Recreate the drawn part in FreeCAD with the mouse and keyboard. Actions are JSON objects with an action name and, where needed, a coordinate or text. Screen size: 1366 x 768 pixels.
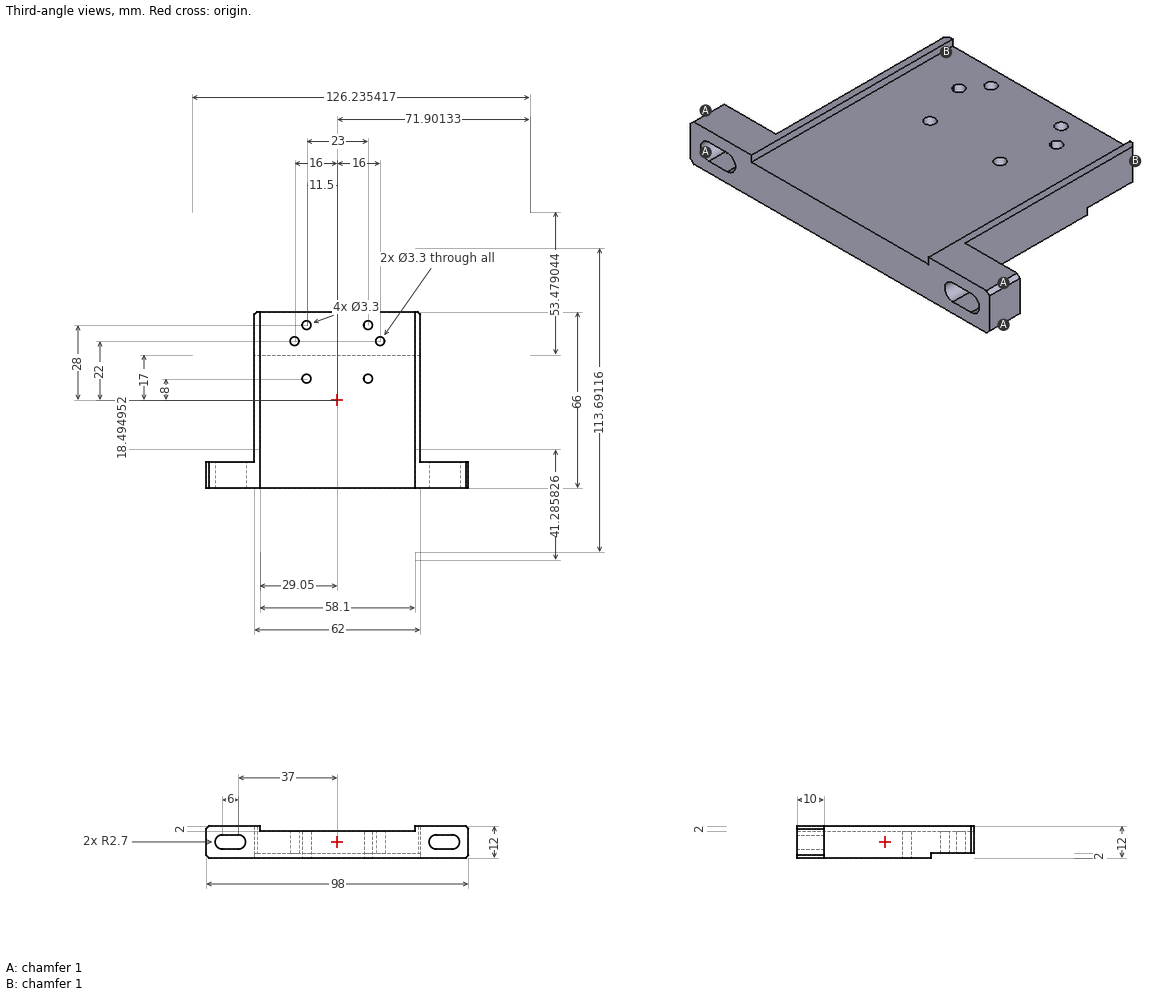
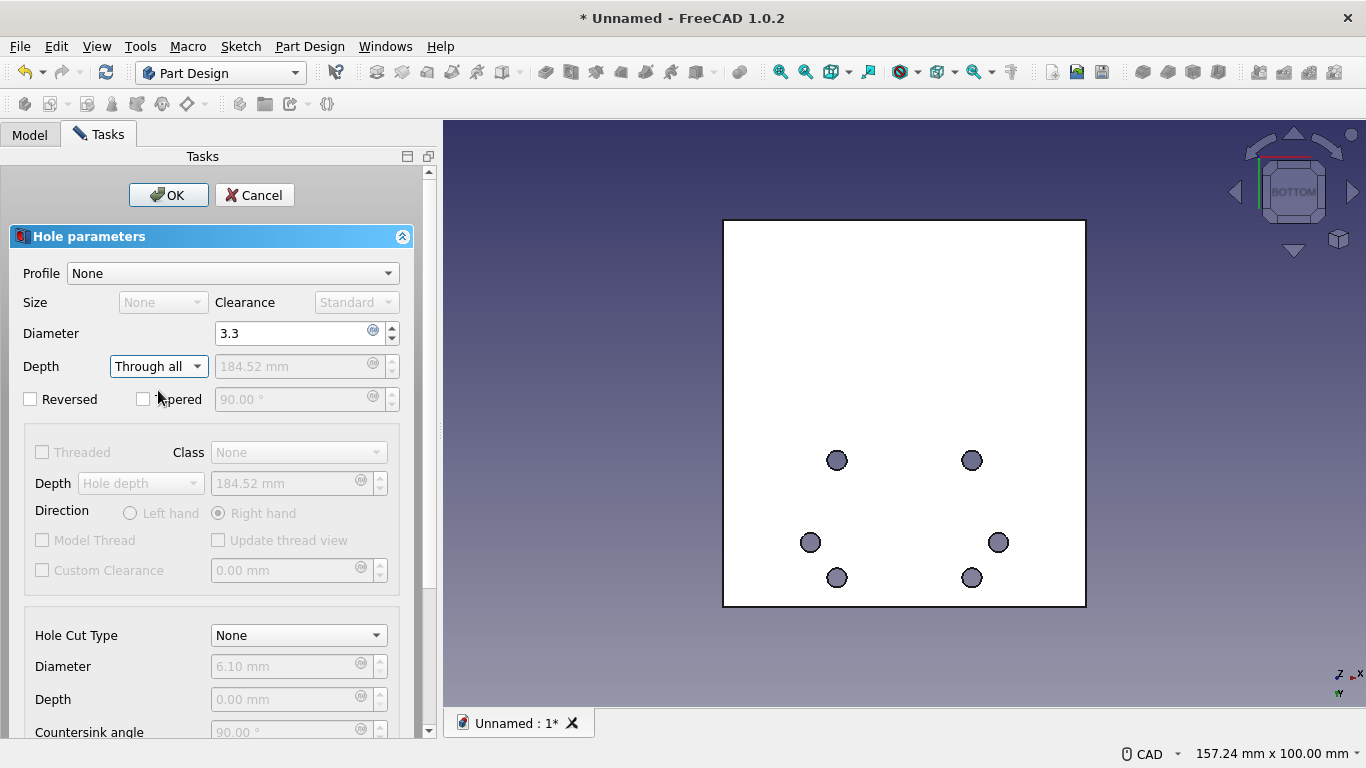
{"action": "left_click", "coordinate": [169, 195]}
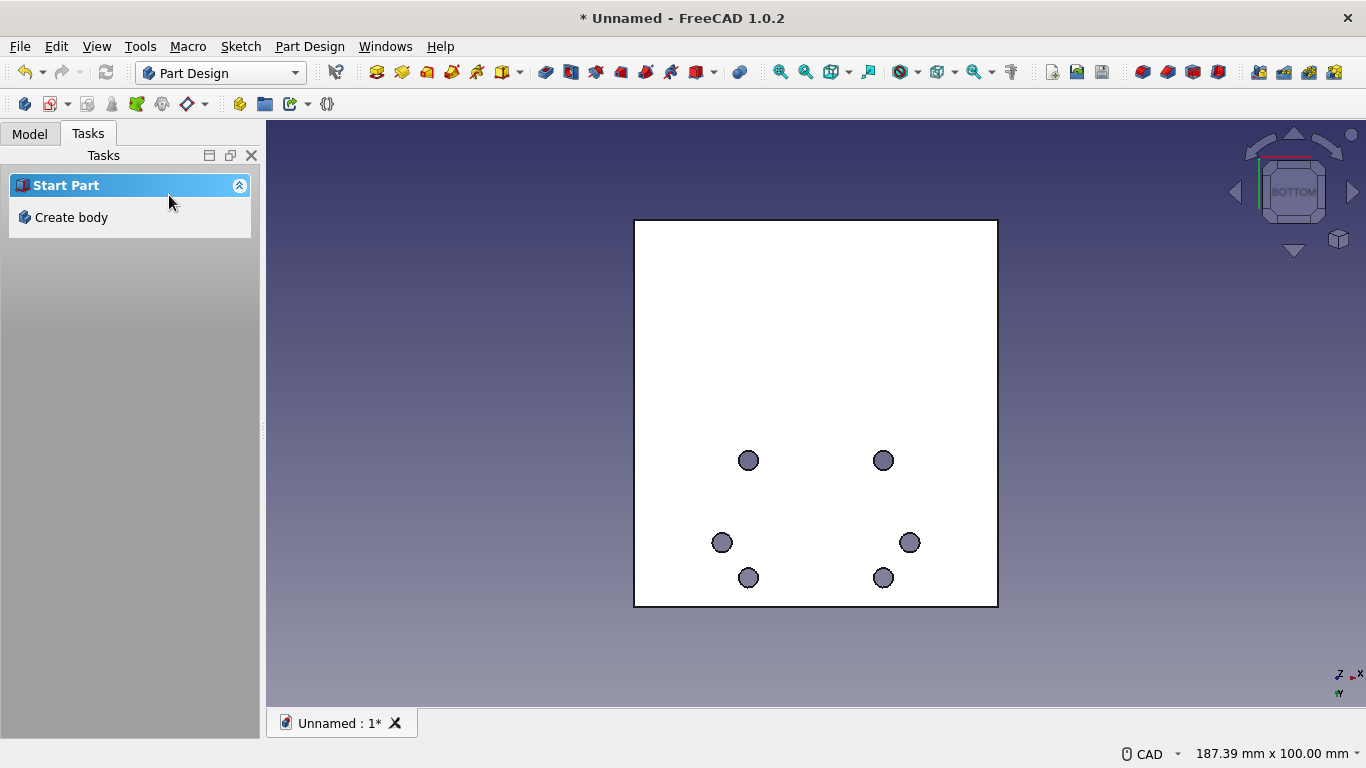
{"action": "key", "text": "0"}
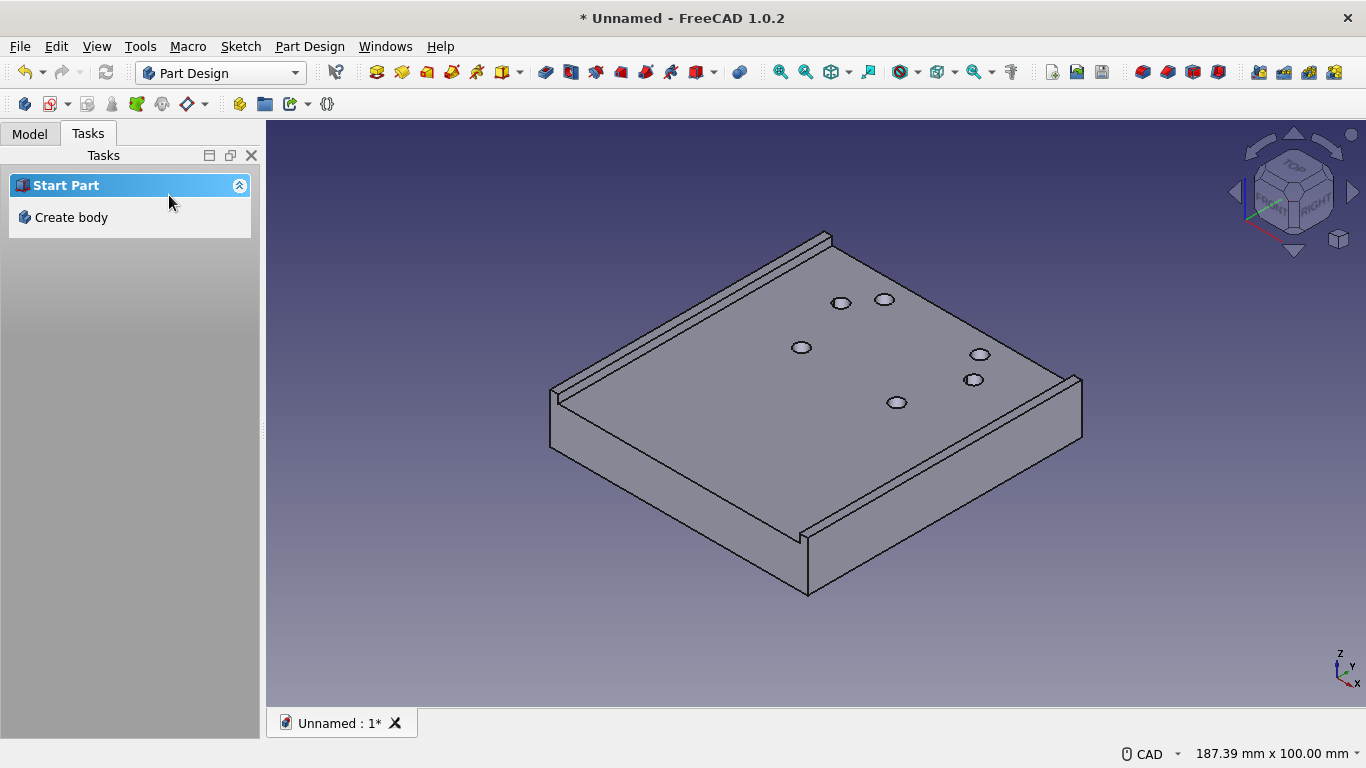
{"action": "left_click", "coordinate": [789, 563]}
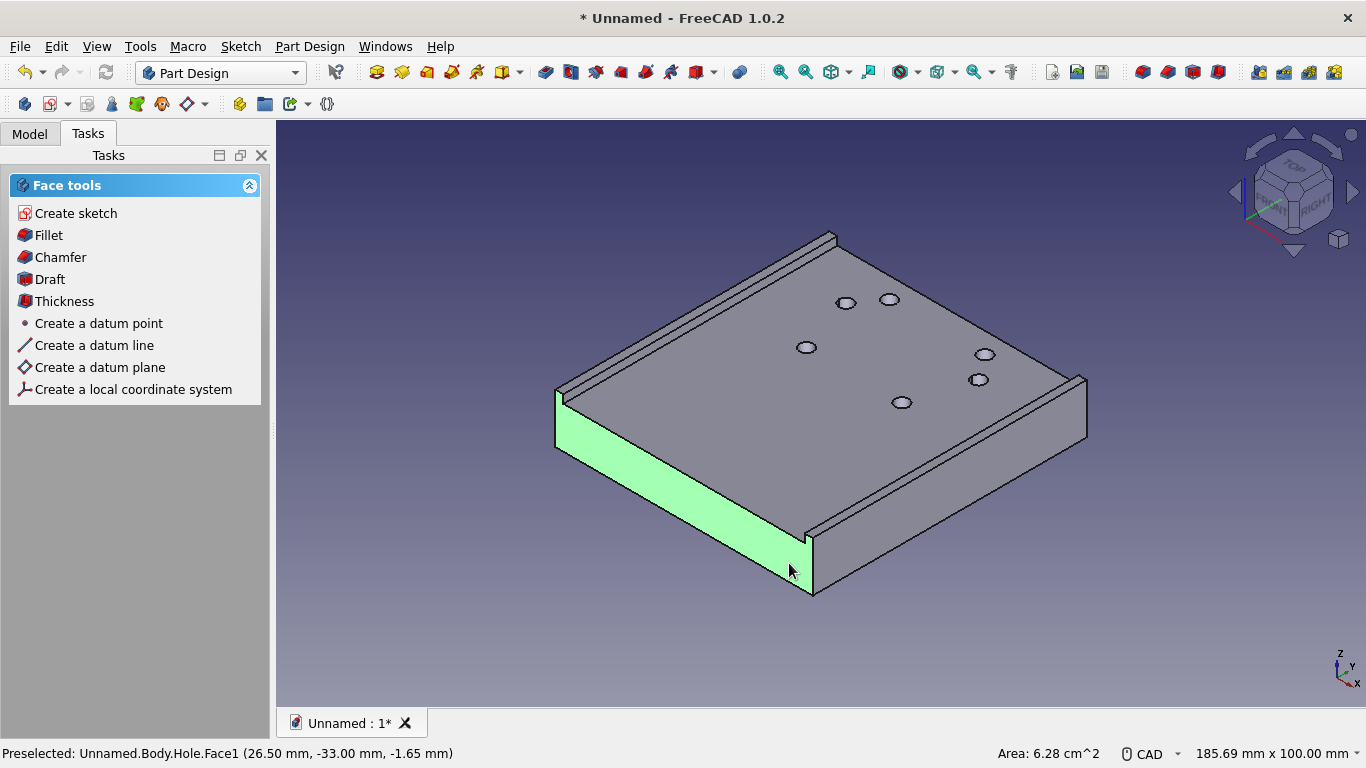
{"action": "left_click", "coordinate": [50, 104]}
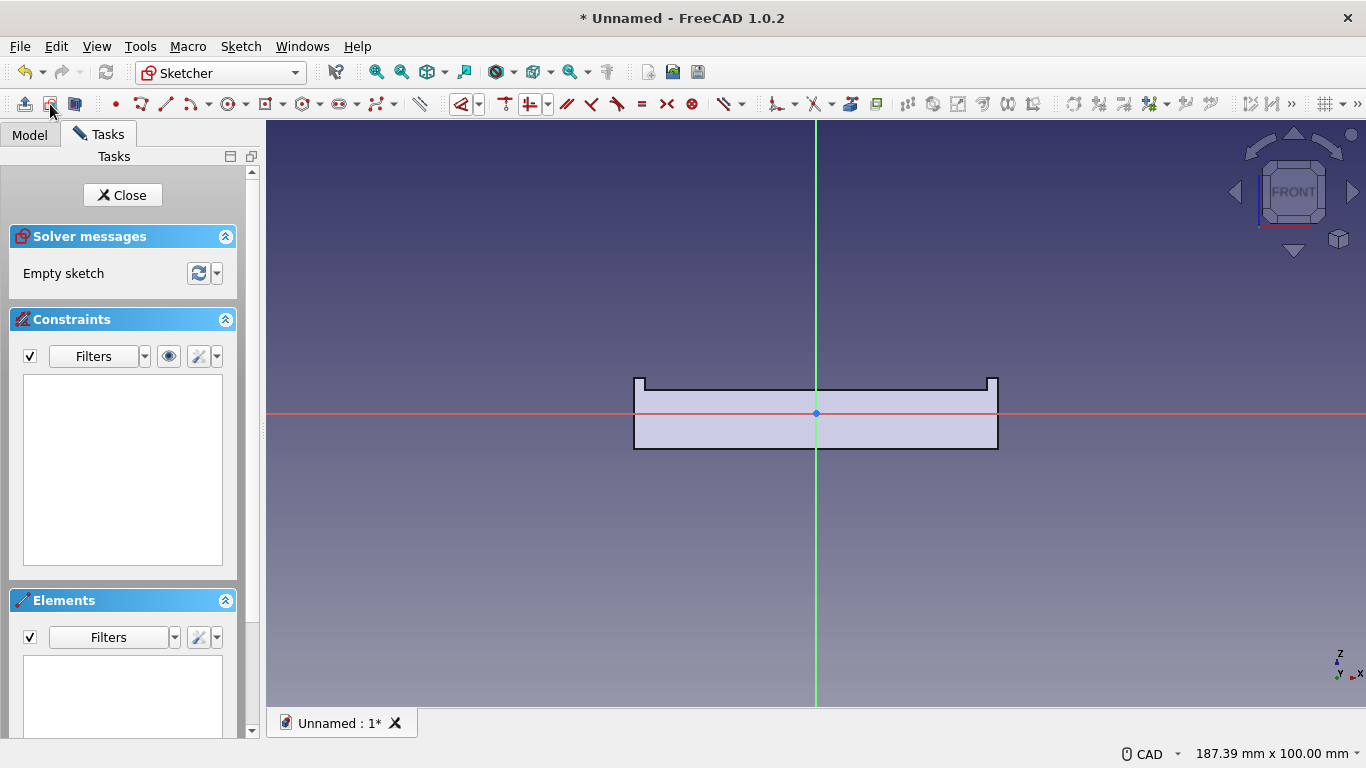
{"action": "left_click", "coordinate": [264, 104]}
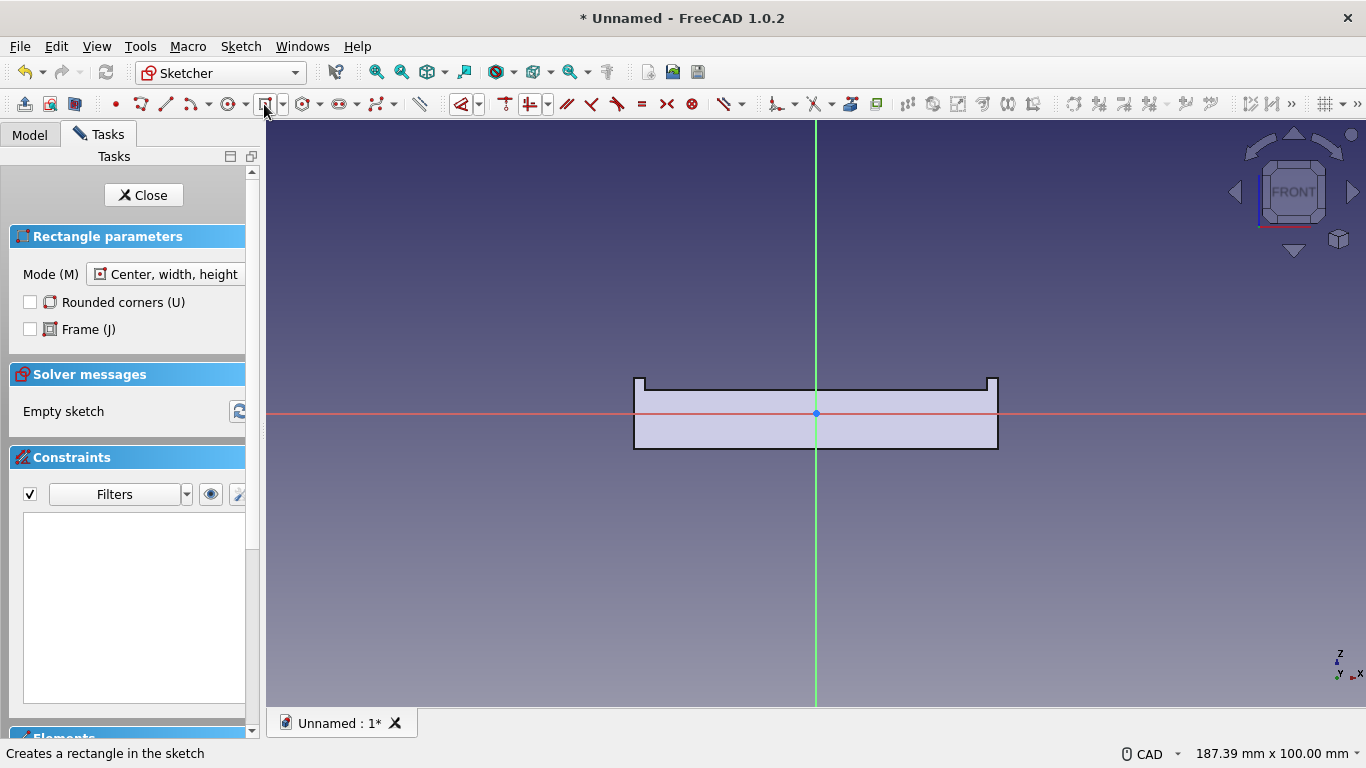
{"action": "left_click", "coordinate": [816, 413]}
{"action": "mouse_move", "coordinate": [1104, 378]}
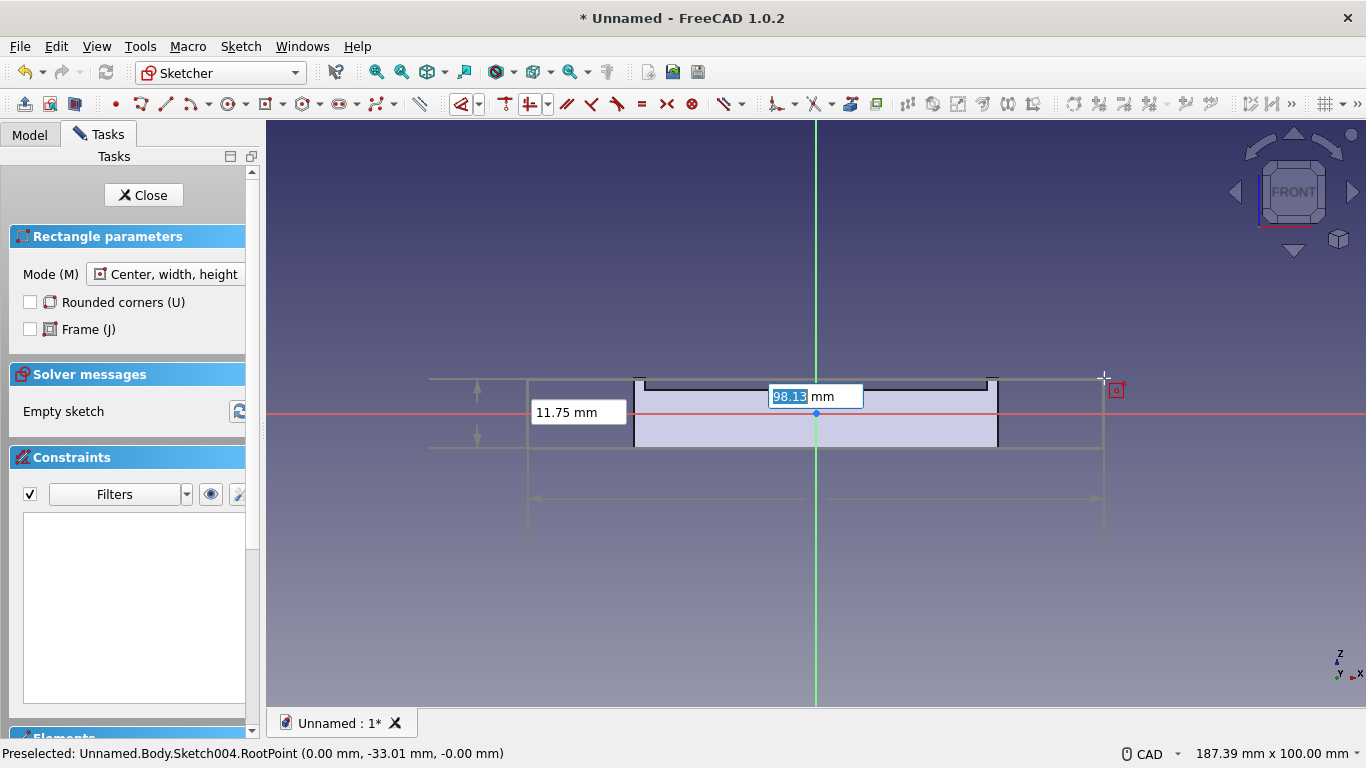
{"action": "type", "text": "98"}
{"action": "key", "text": "Tab"}
{"action": "type", "text": "12"}
{"action": "key", "text": "Return"}
{"action": "key", "text": "Escape"}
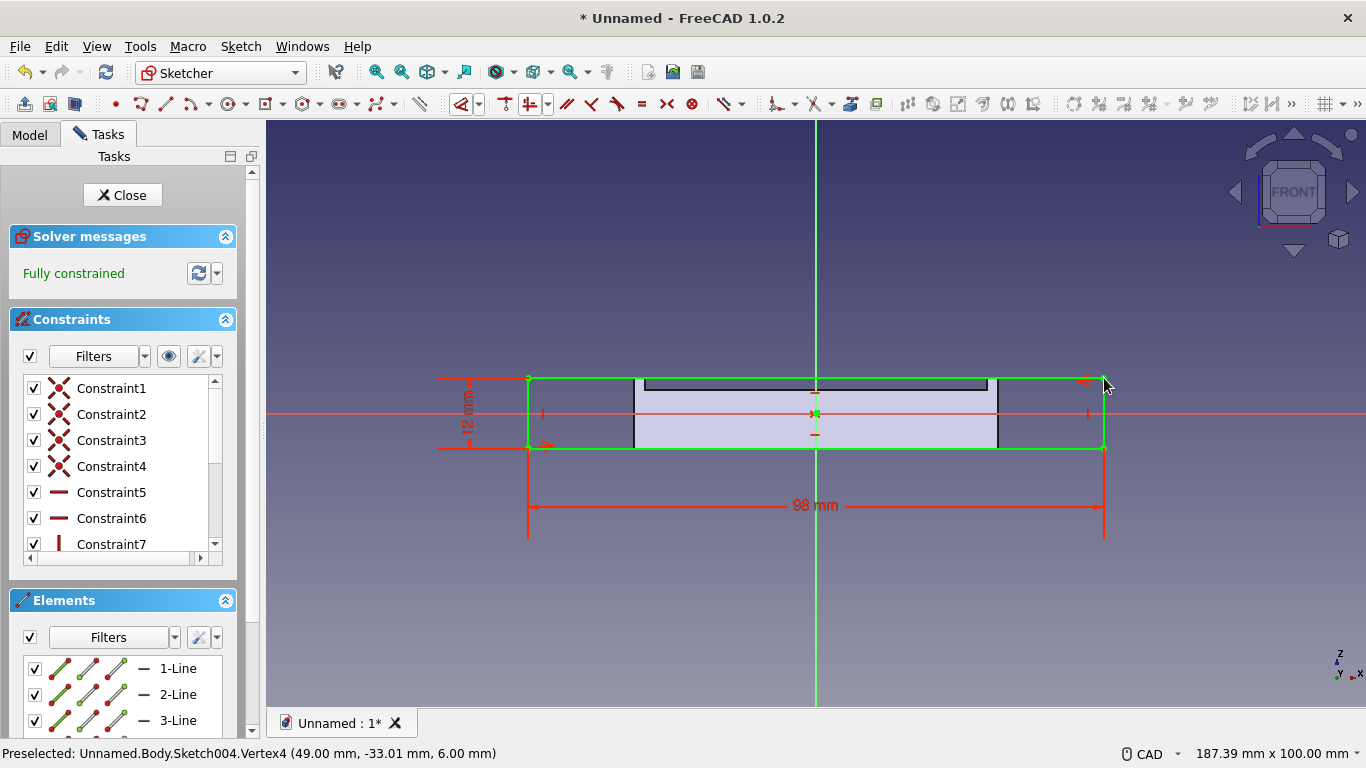
{"action": "left_click", "coordinate": [123, 195]}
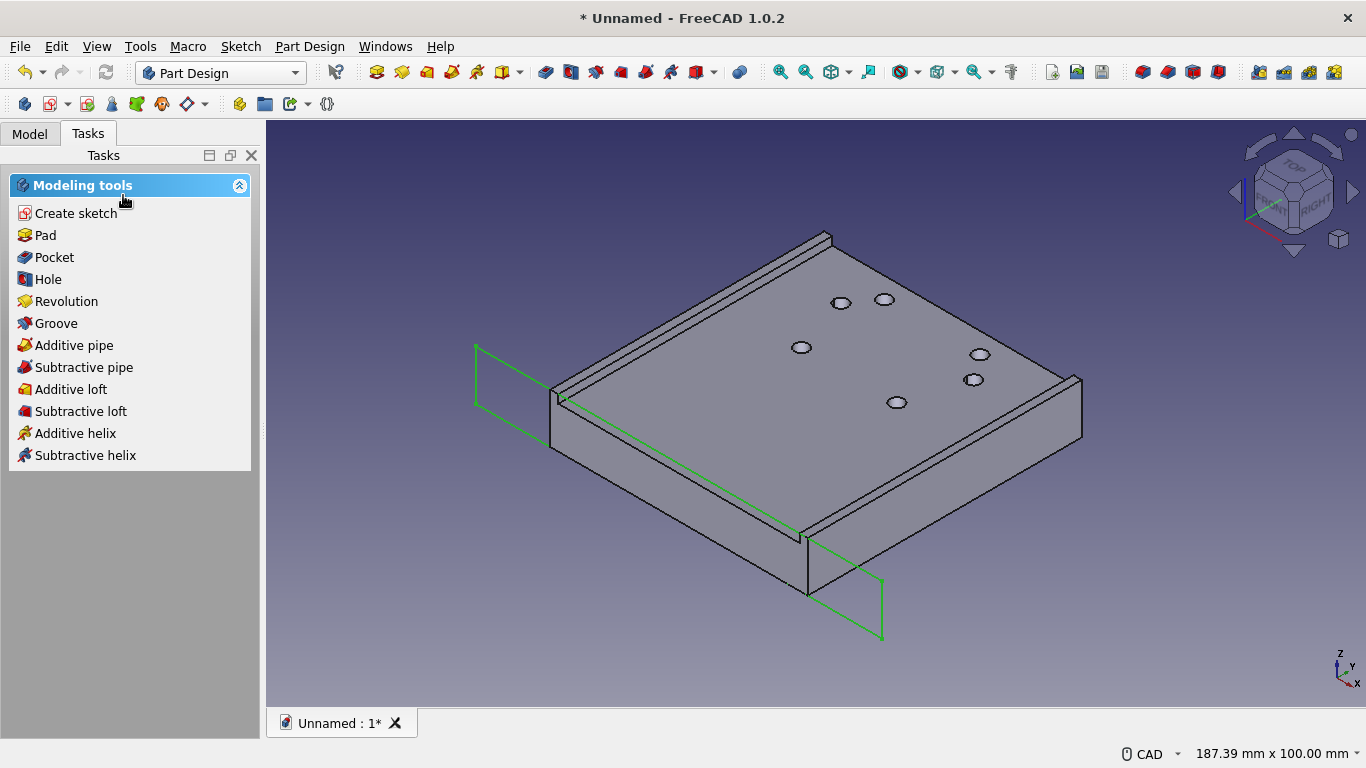
{"action": "left_click", "coordinate": [377, 72]}